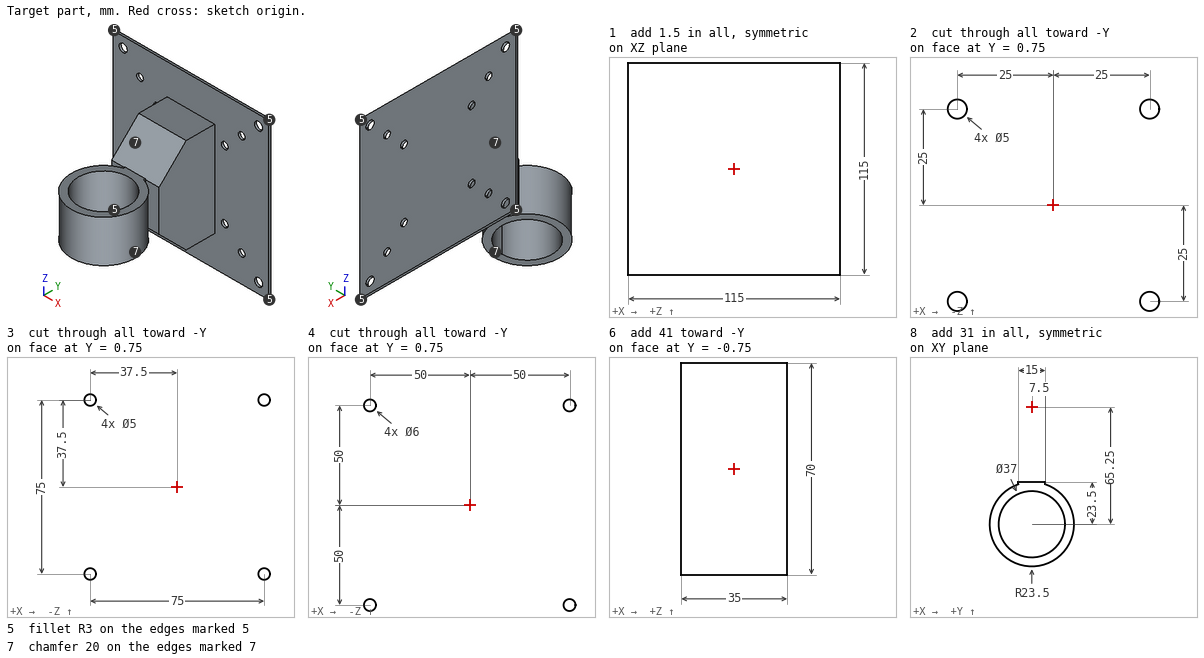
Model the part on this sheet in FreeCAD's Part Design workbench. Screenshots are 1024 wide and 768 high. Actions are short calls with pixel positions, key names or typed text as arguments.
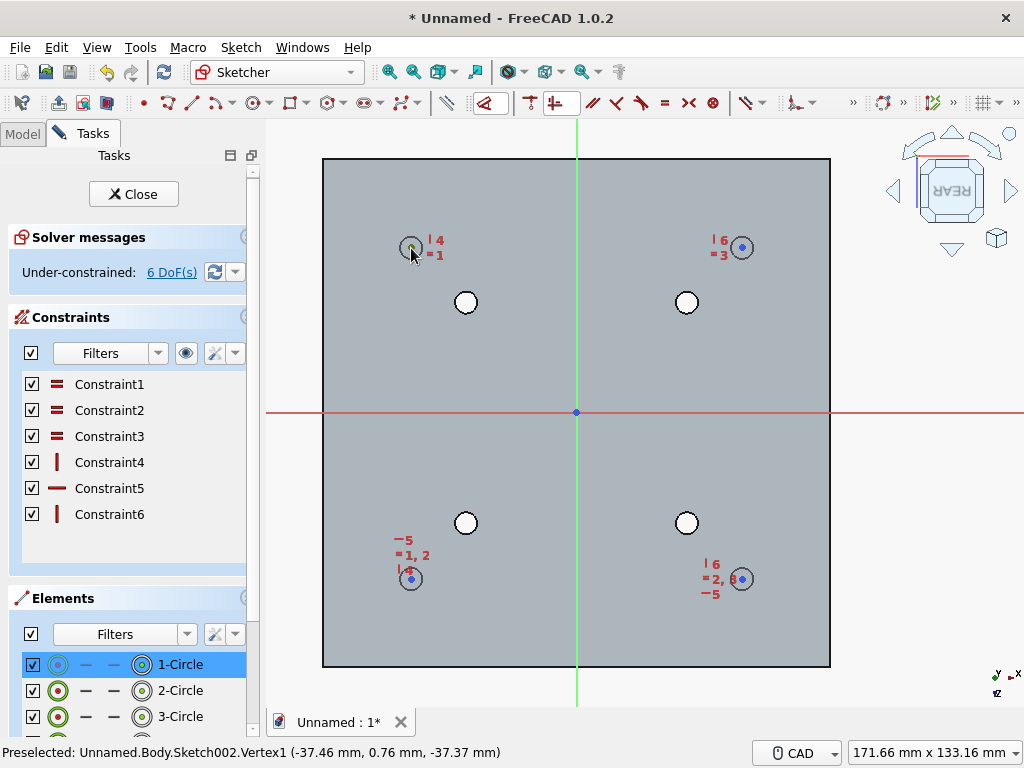
click(742, 248)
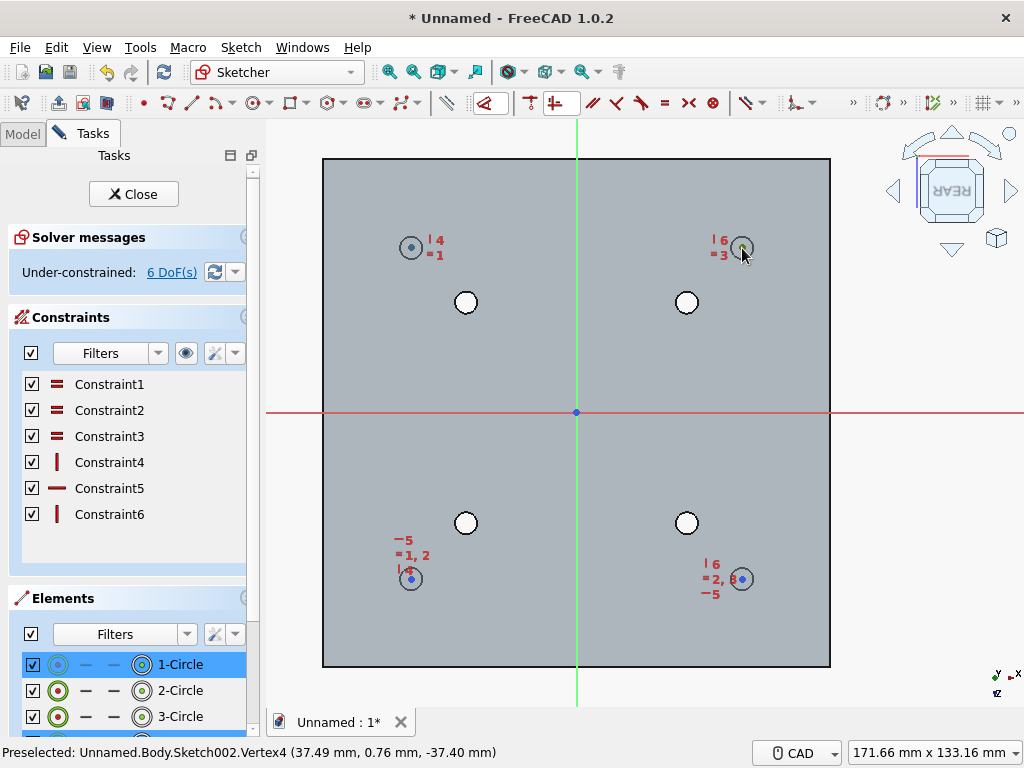
click(574, 104)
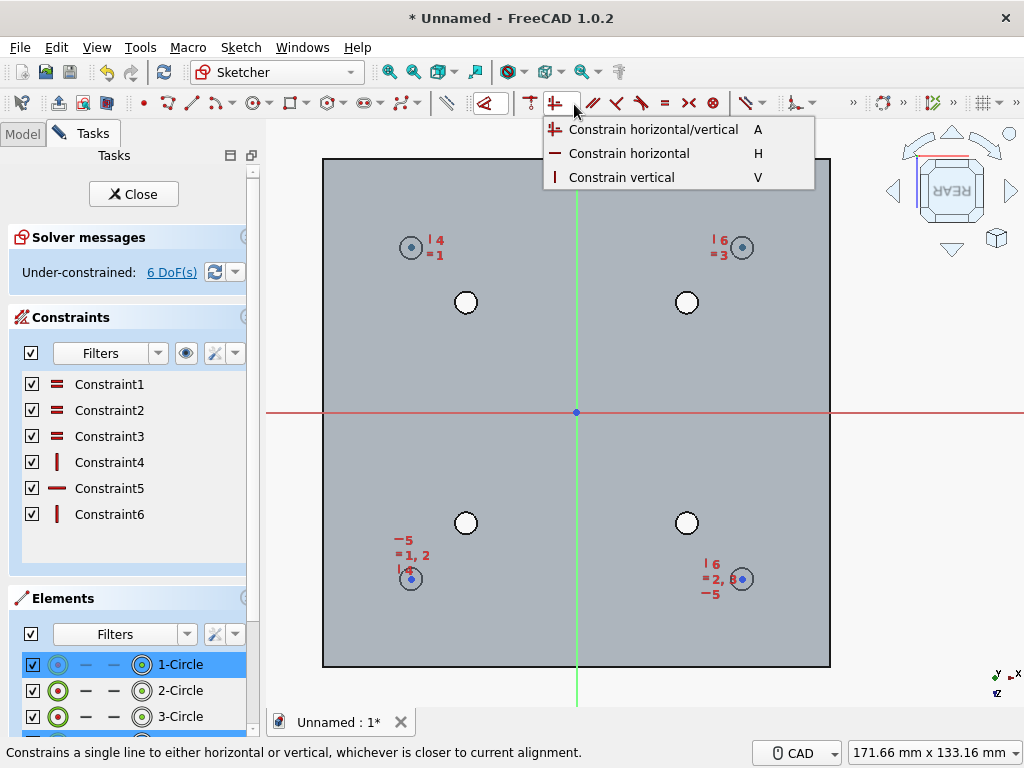
click(679, 153)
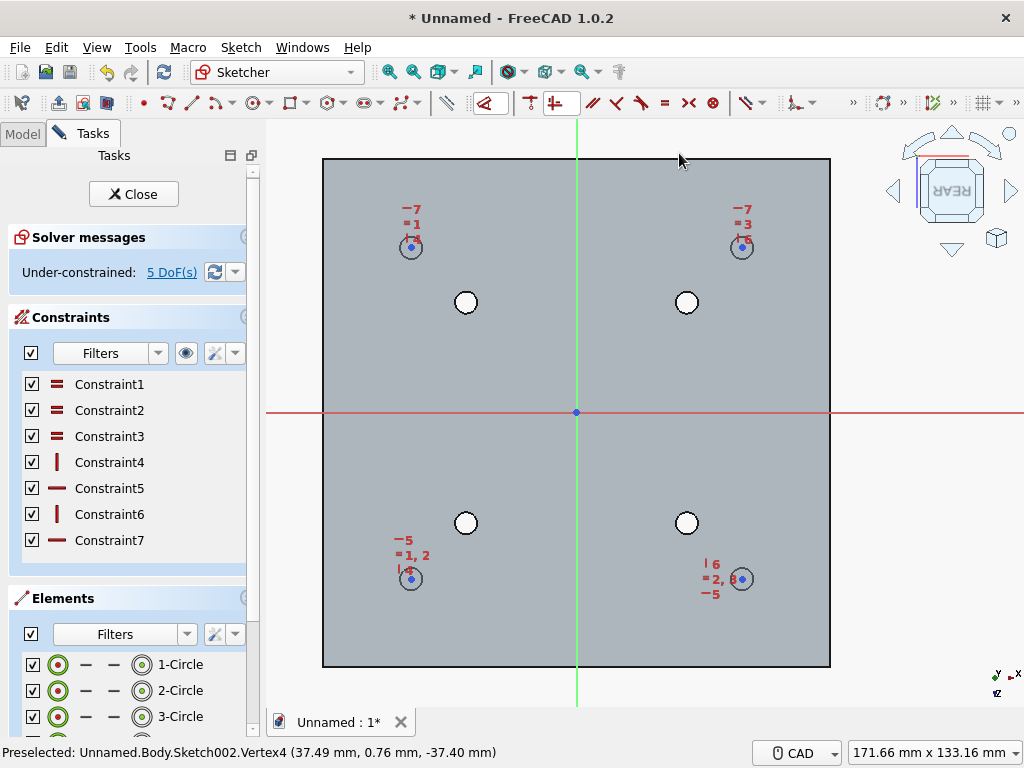
key(d)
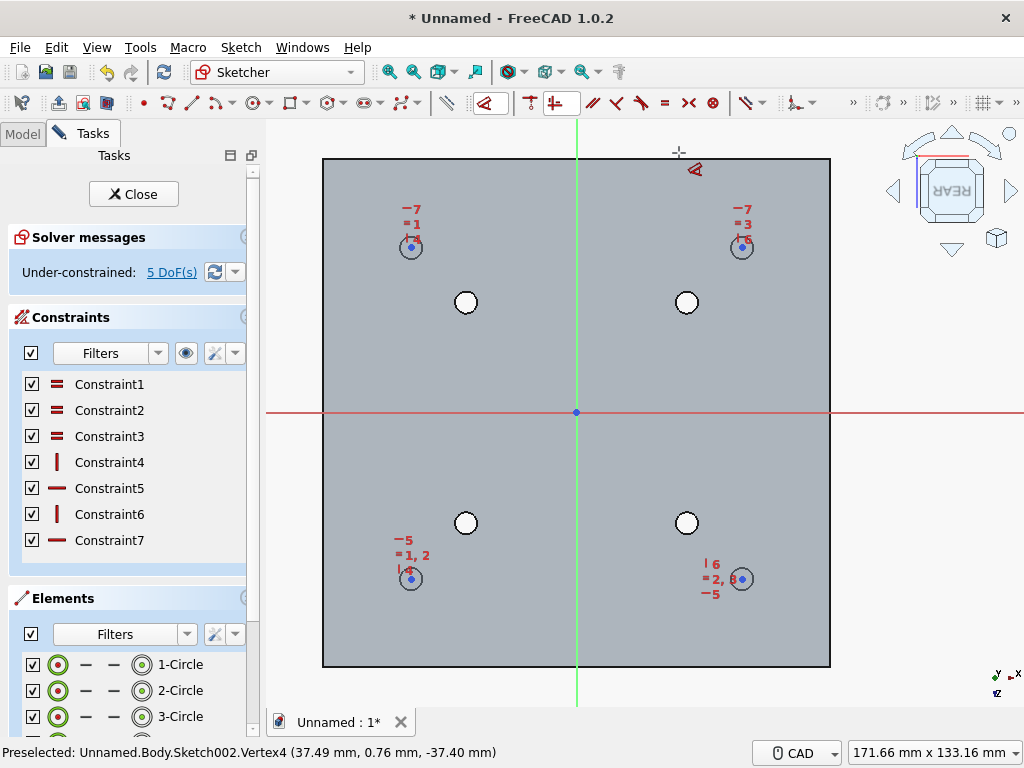
scroll(419, 240, up, 3)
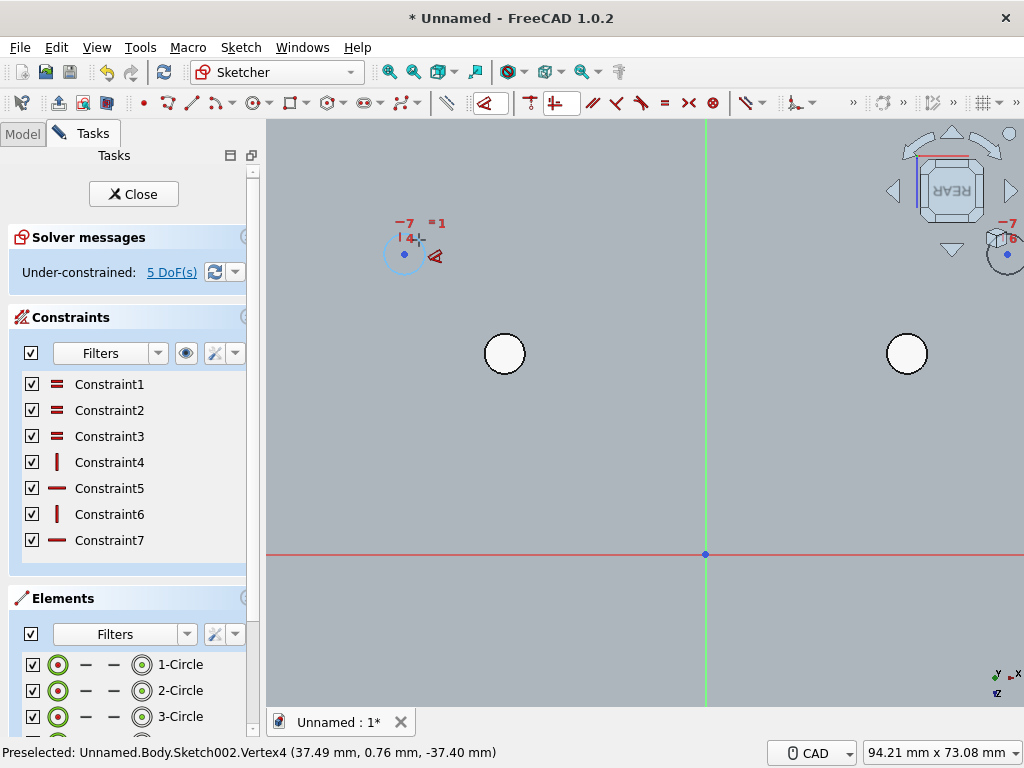
click(419, 240)
click(442, 218)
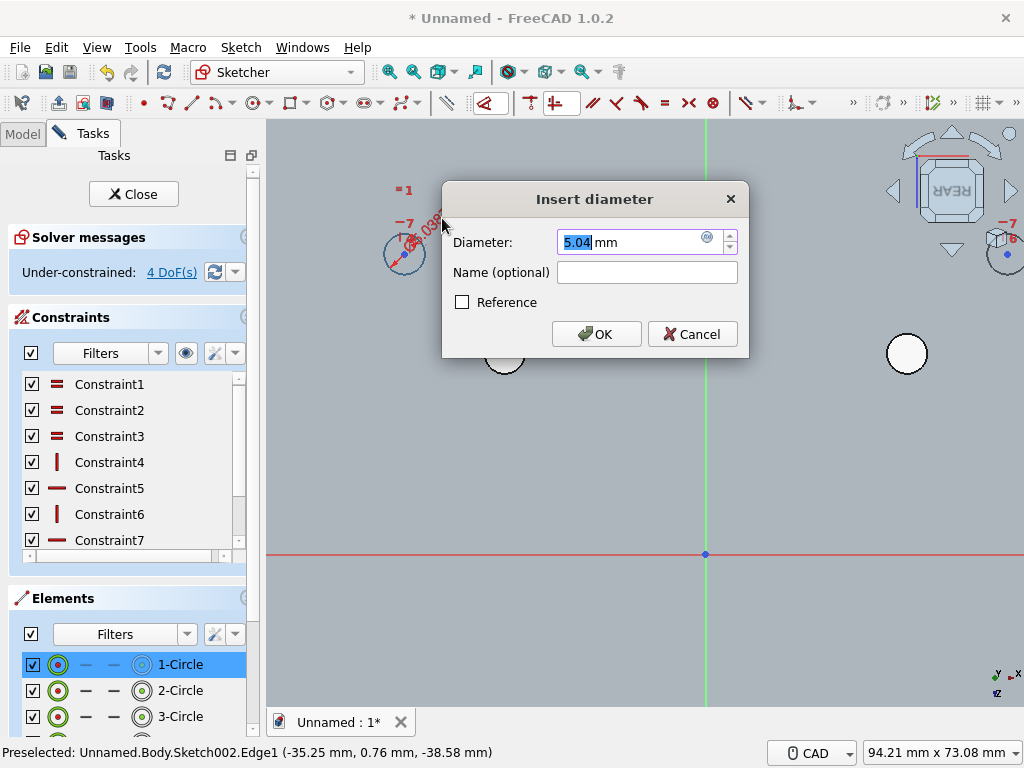
text(5)
key(Return)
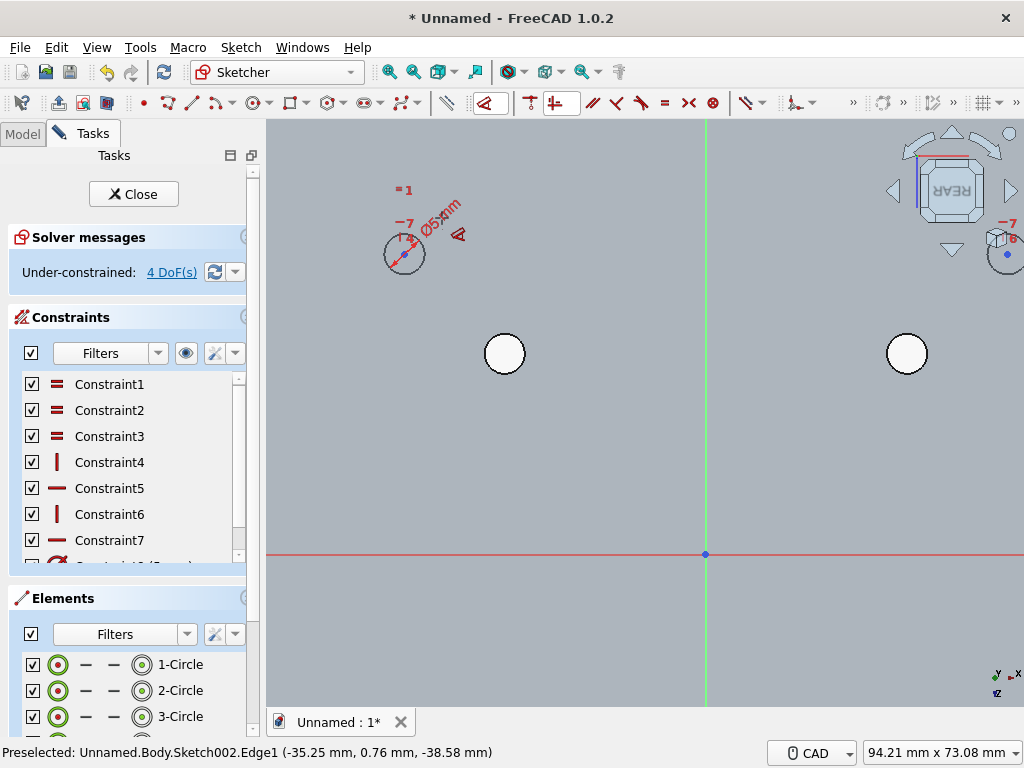
click(405, 254)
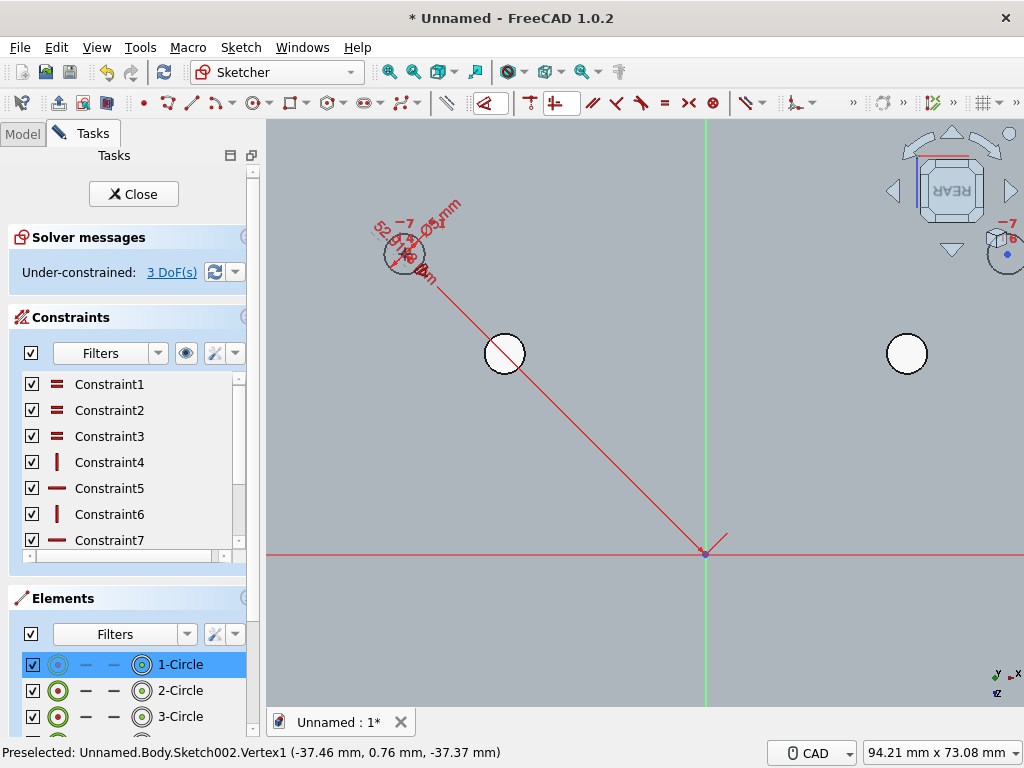
scroll(419, 240, down, 3)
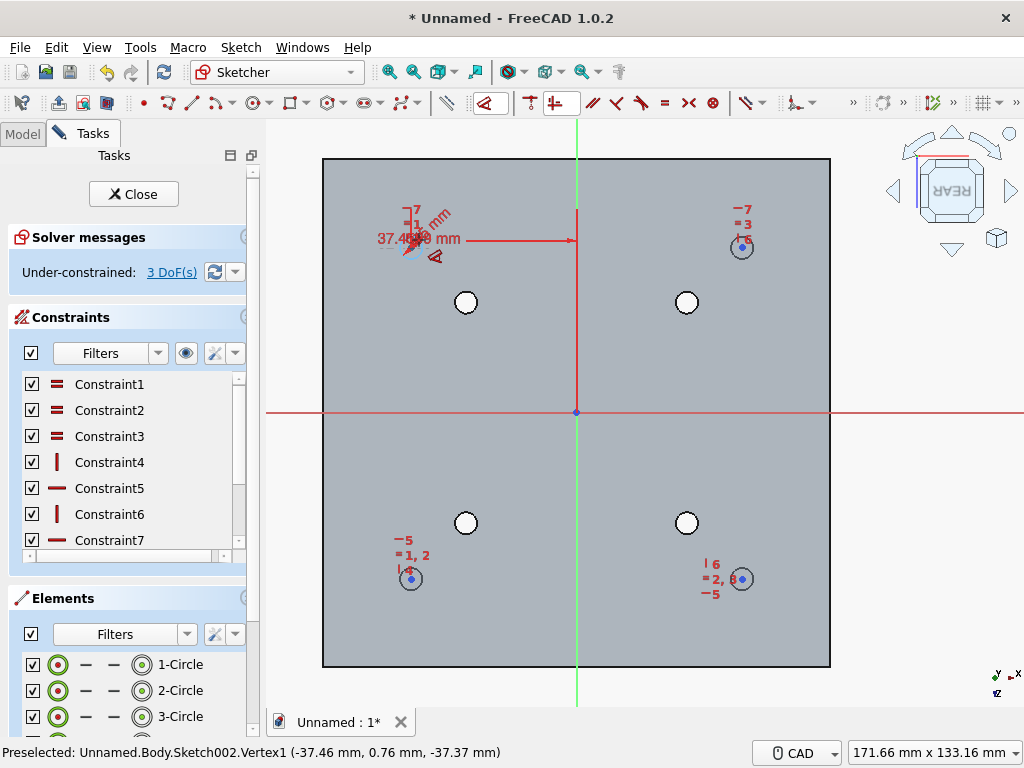
click(411, 579)
click(377, 337)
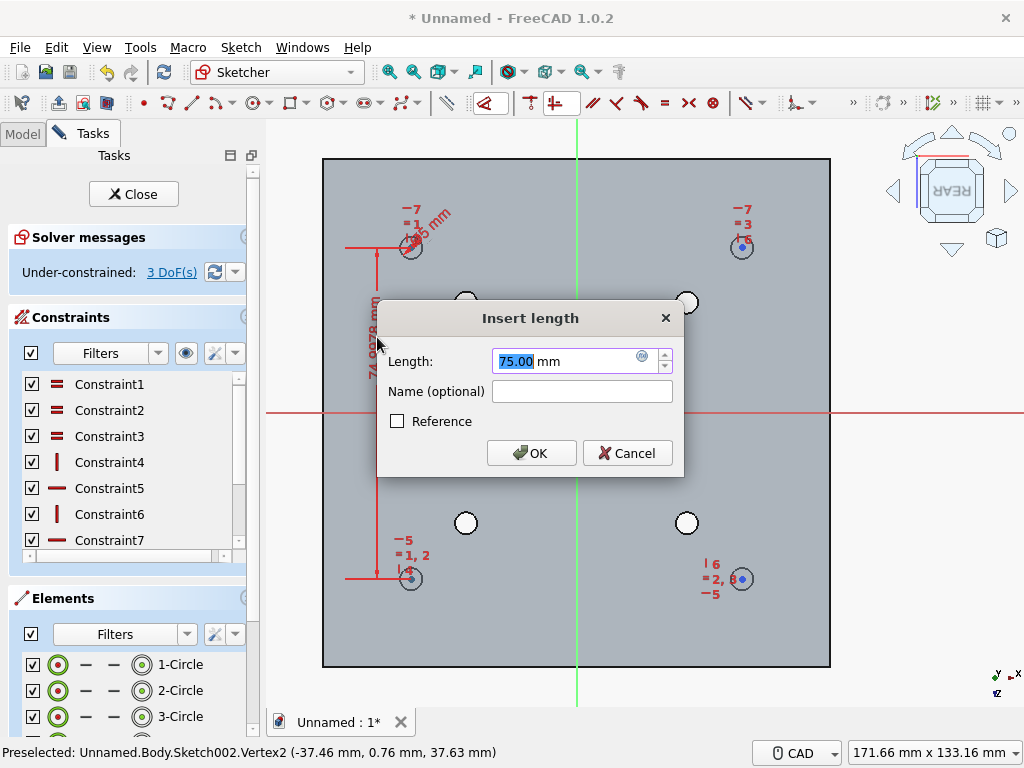
text(75)
key(Return)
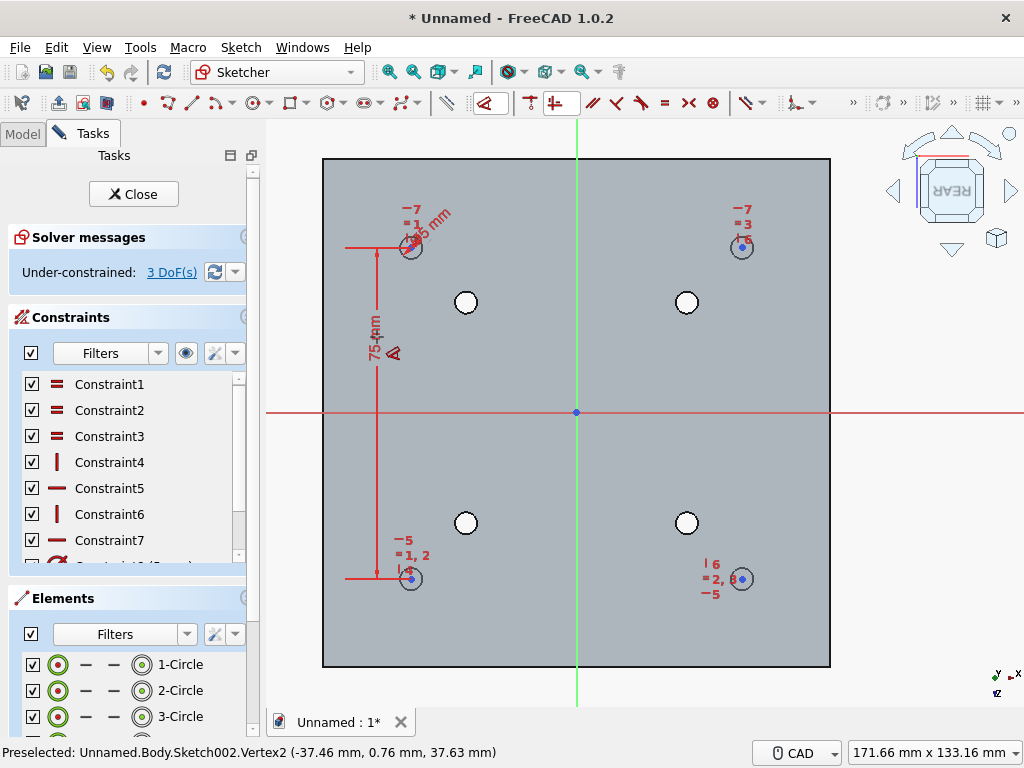
click(411, 579)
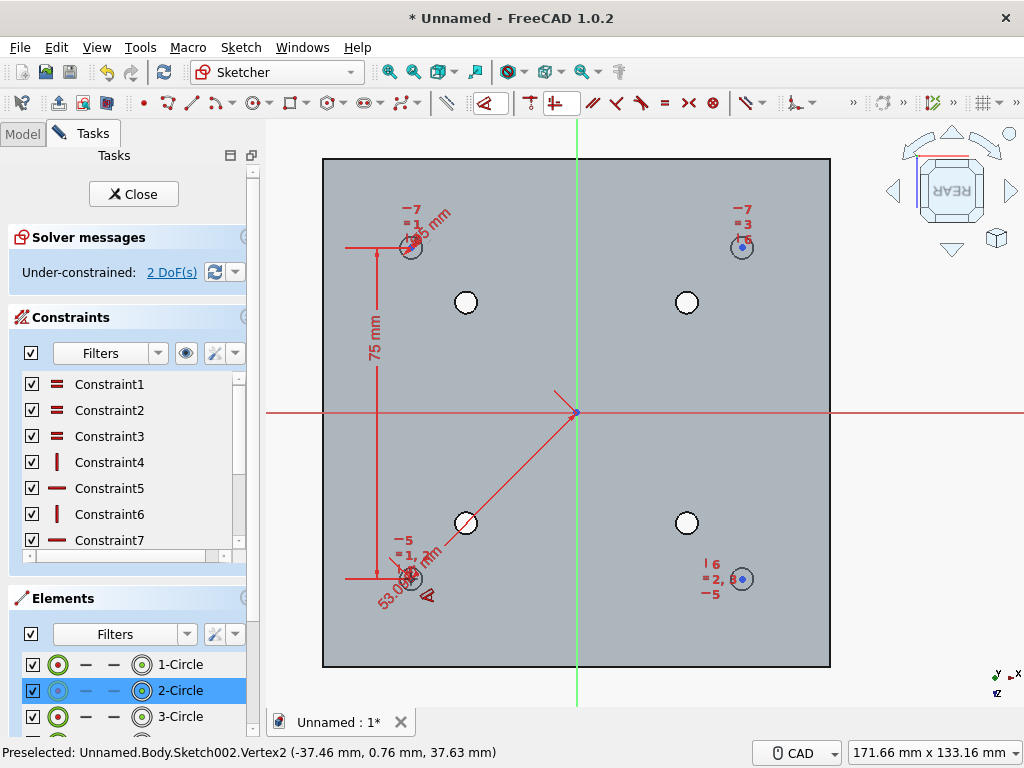
click(742, 579)
click(501, 613)